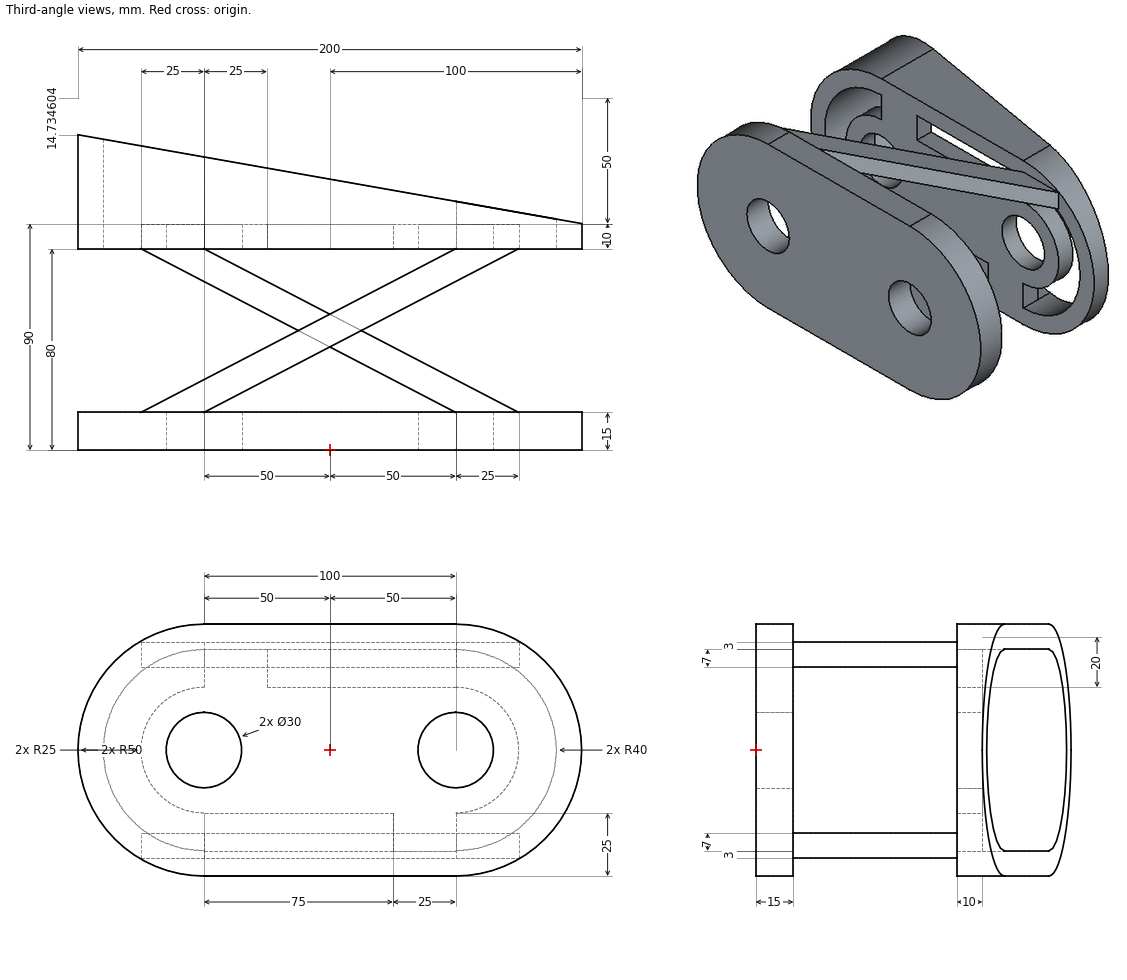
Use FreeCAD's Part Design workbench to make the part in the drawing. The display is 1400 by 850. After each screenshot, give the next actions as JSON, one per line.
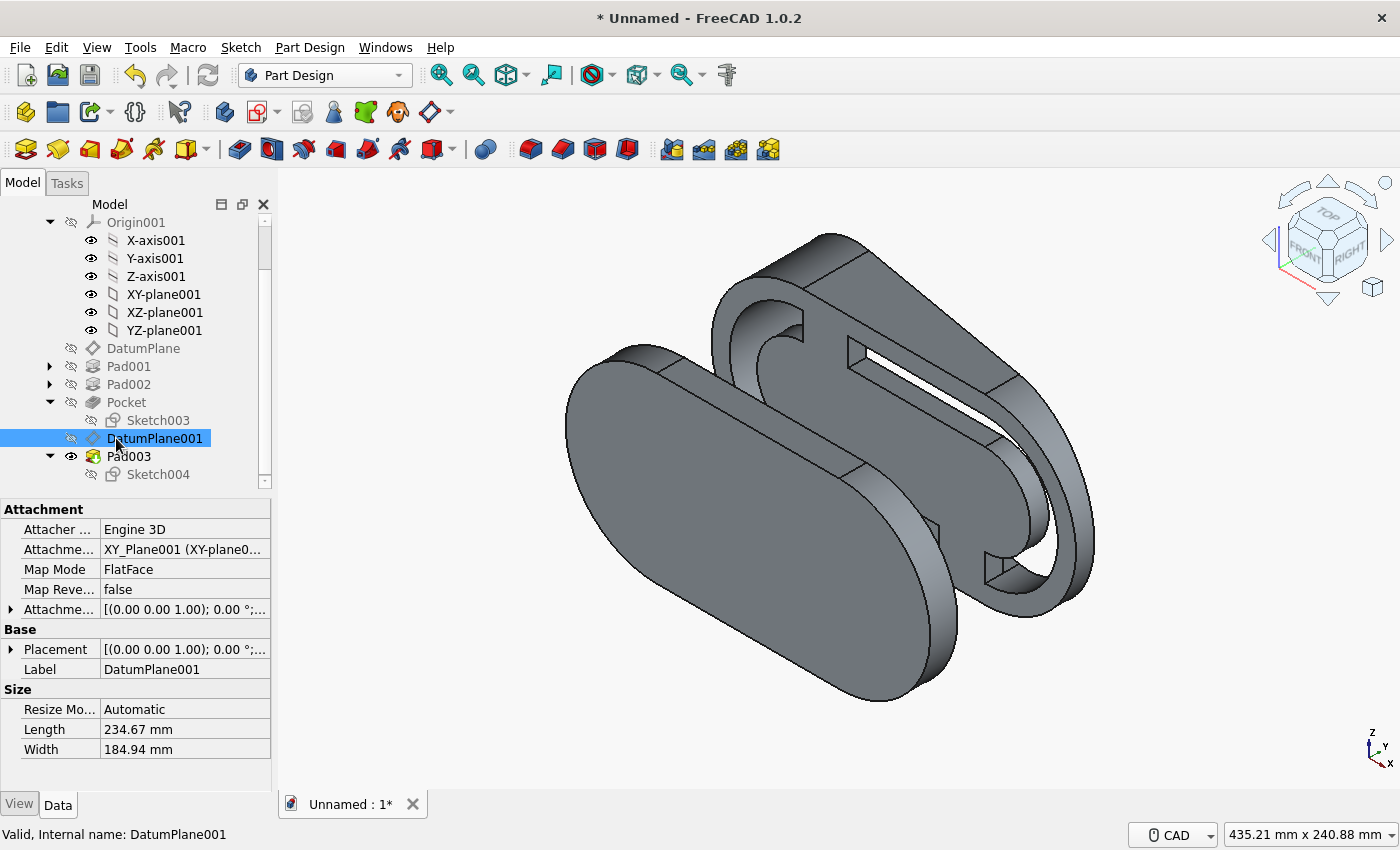
{"action": "scroll", "coordinate": [140, 344], "scroll_direction": "down", "scroll_amount": 3}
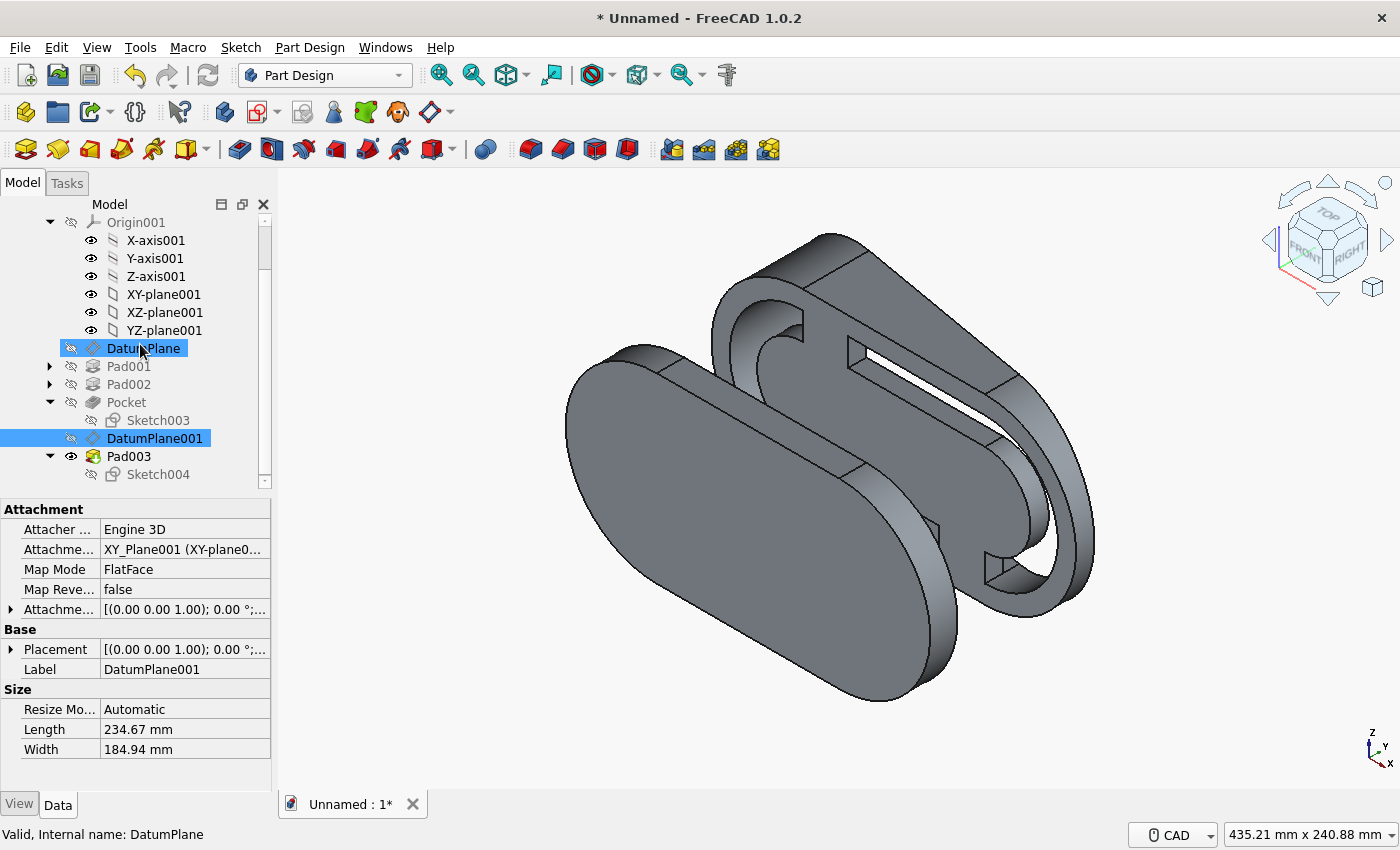
{"action": "scroll", "coordinate": [140, 344], "scroll_direction": "up", "scroll_amount": 15}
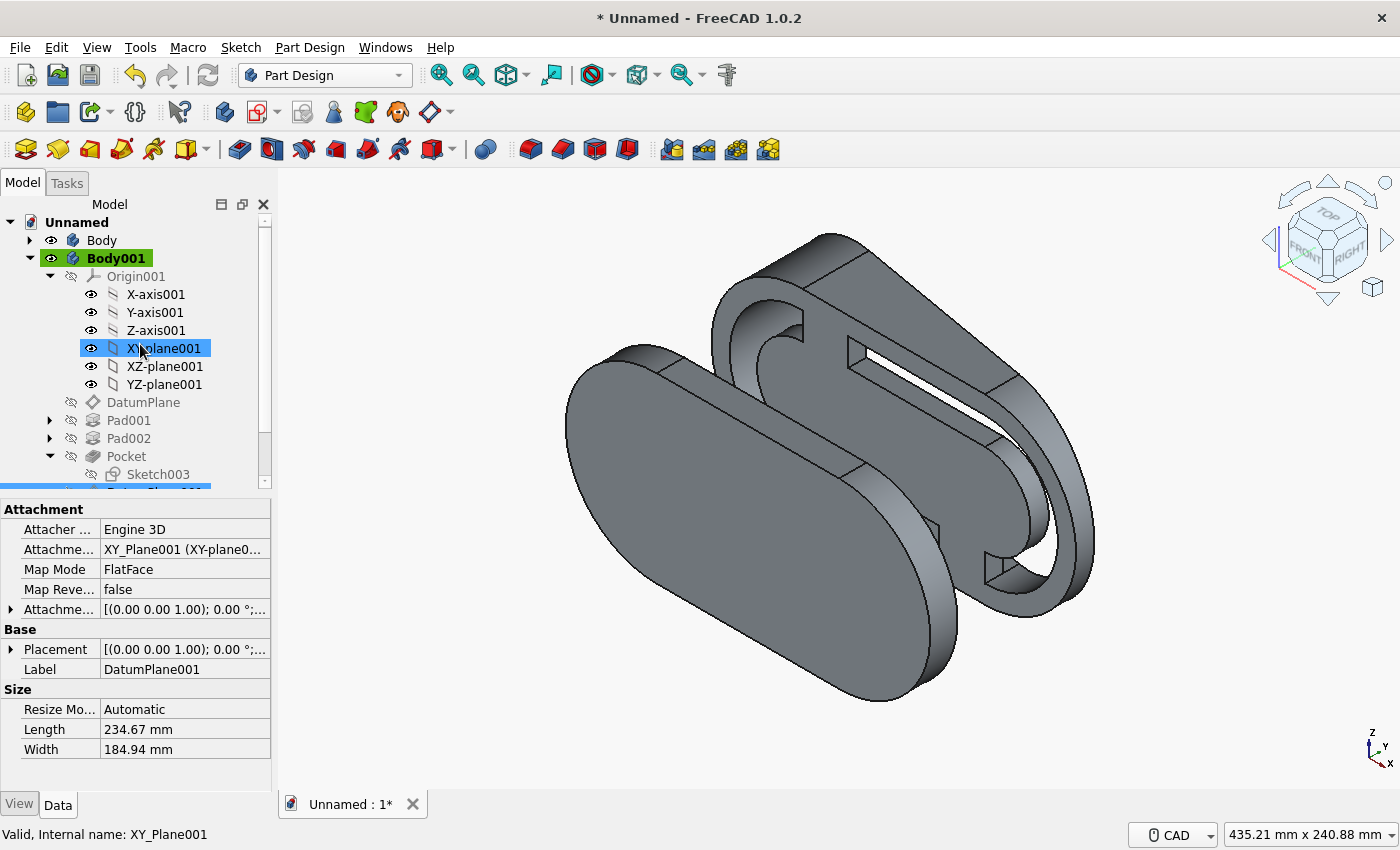
{"action": "double_click", "coordinate": [96, 240]}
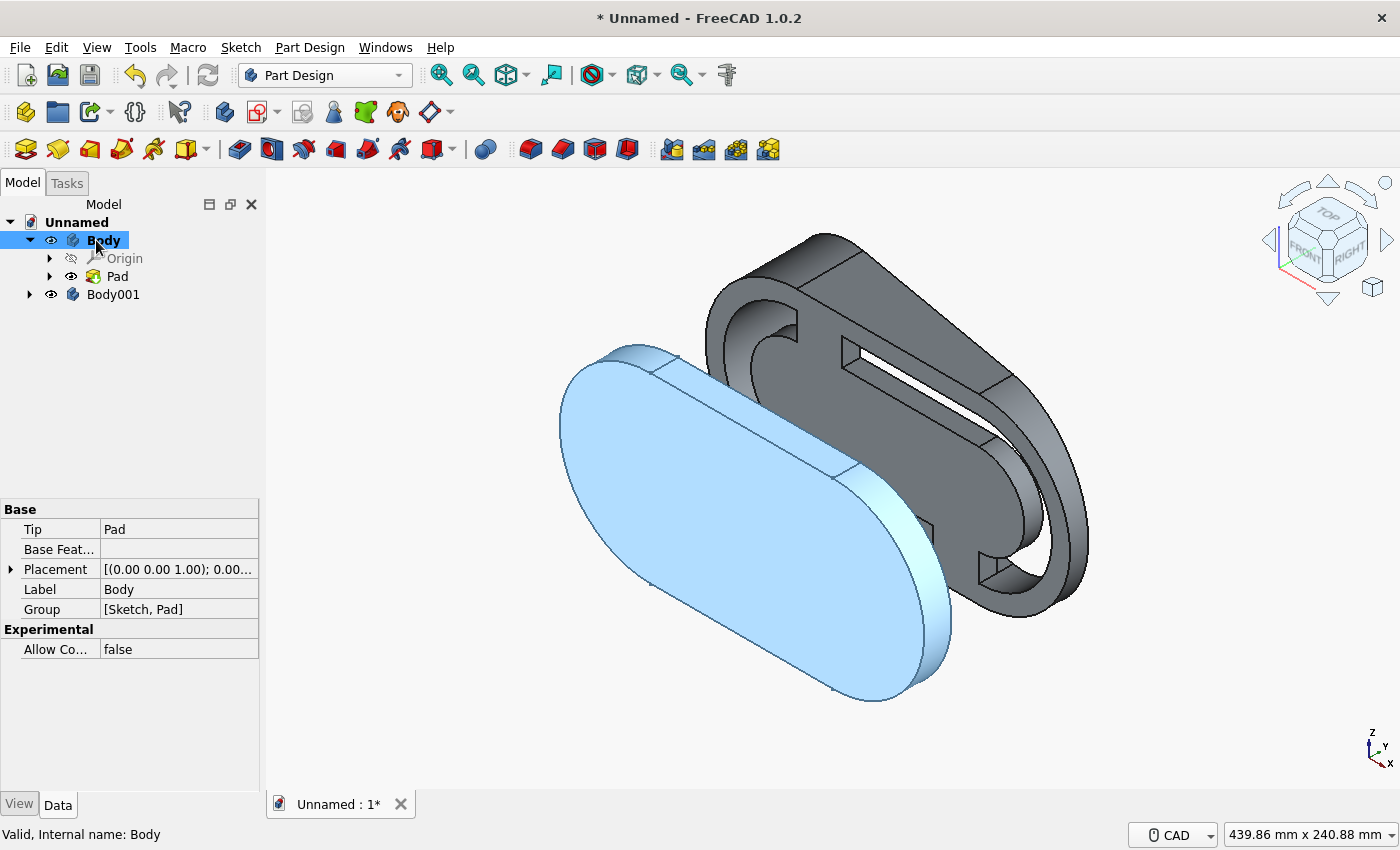
{"action": "left_click", "coordinate": [96, 240]}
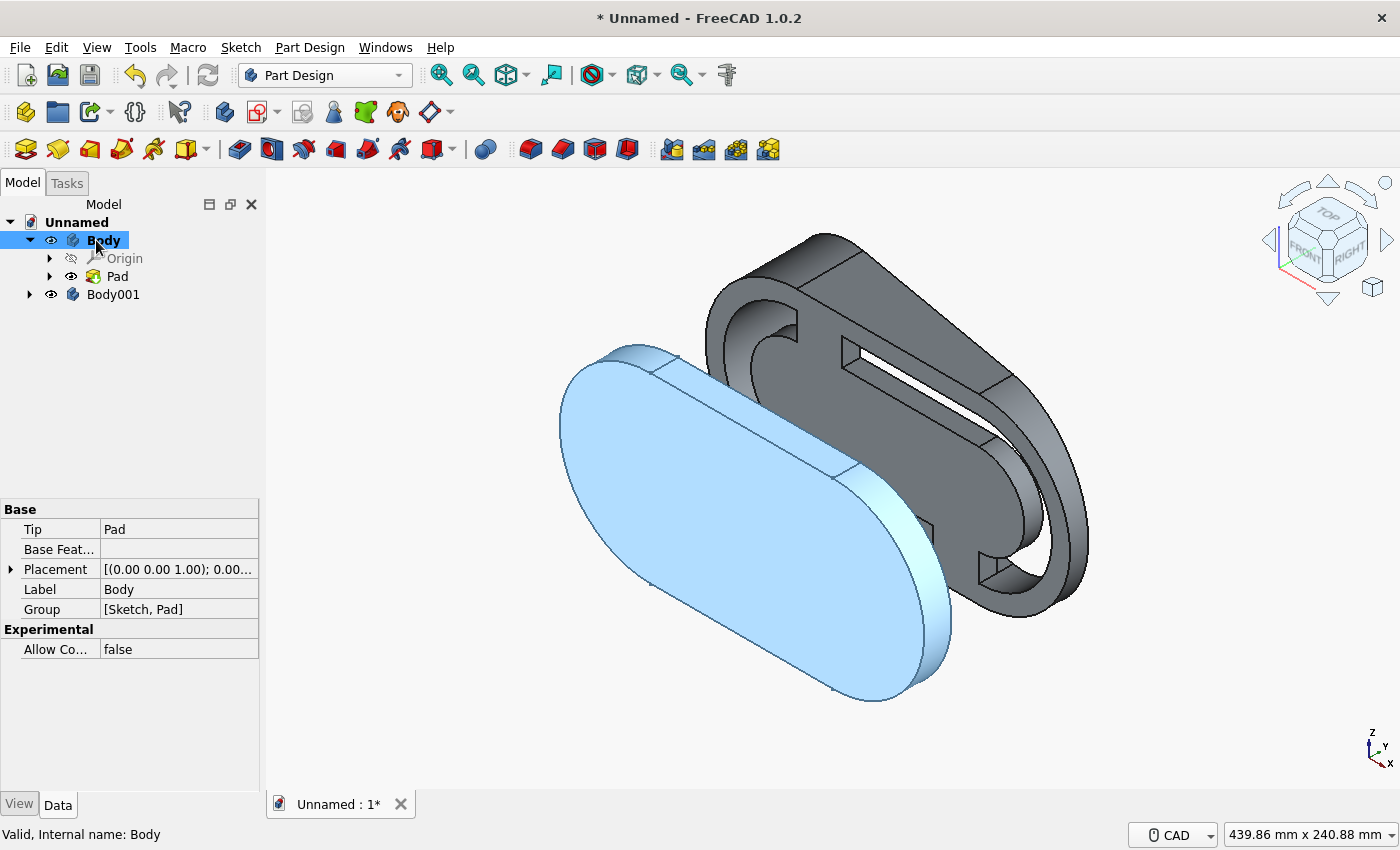
{"action": "left_click", "coordinate": [146, 649]}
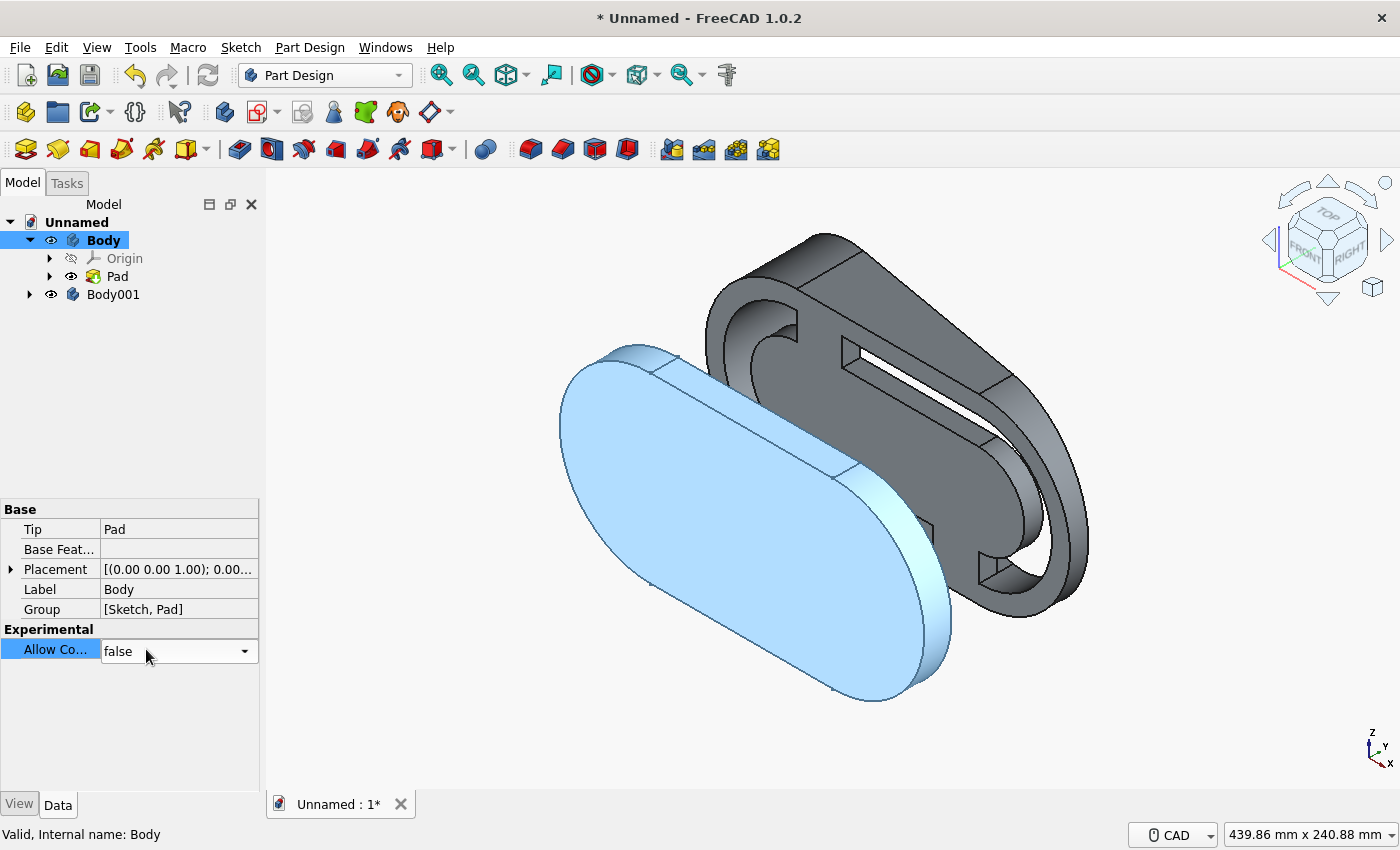
{"action": "left_click", "coordinate": [146, 649]}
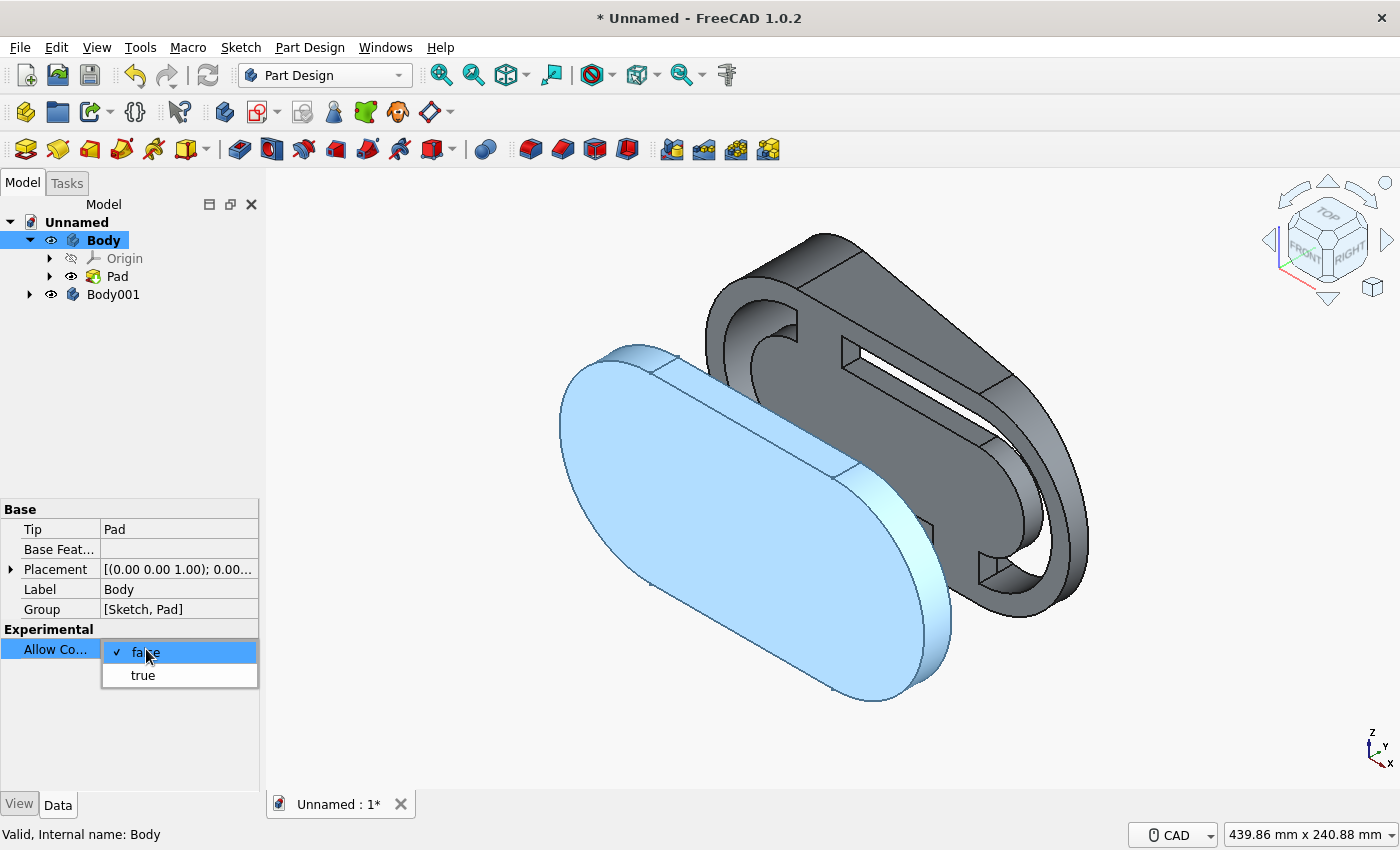
{"action": "left_click", "coordinate": [179, 676]}
{"action": "key", "text": "Return"}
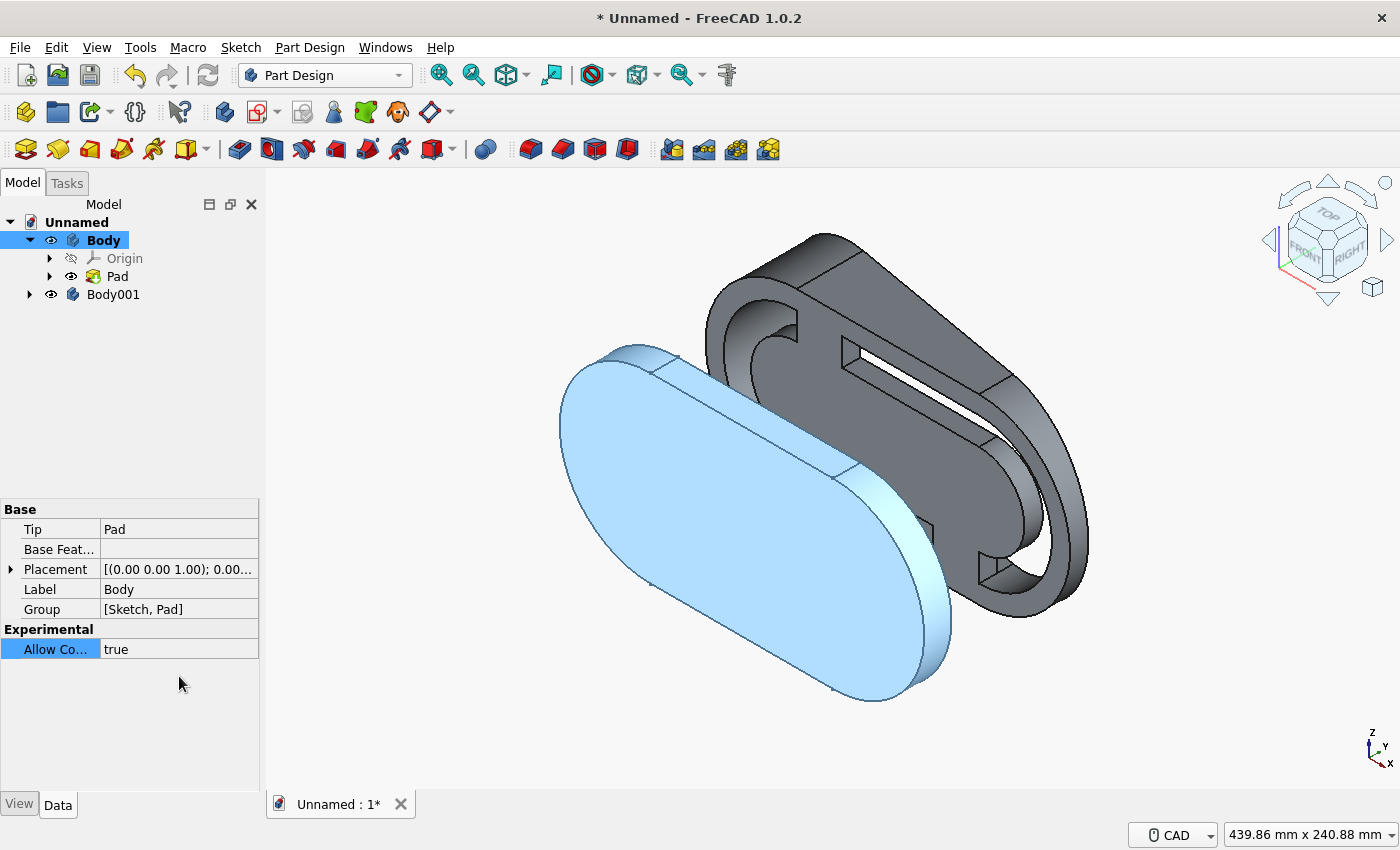
{"action": "left_click", "coordinate": [96, 294]}